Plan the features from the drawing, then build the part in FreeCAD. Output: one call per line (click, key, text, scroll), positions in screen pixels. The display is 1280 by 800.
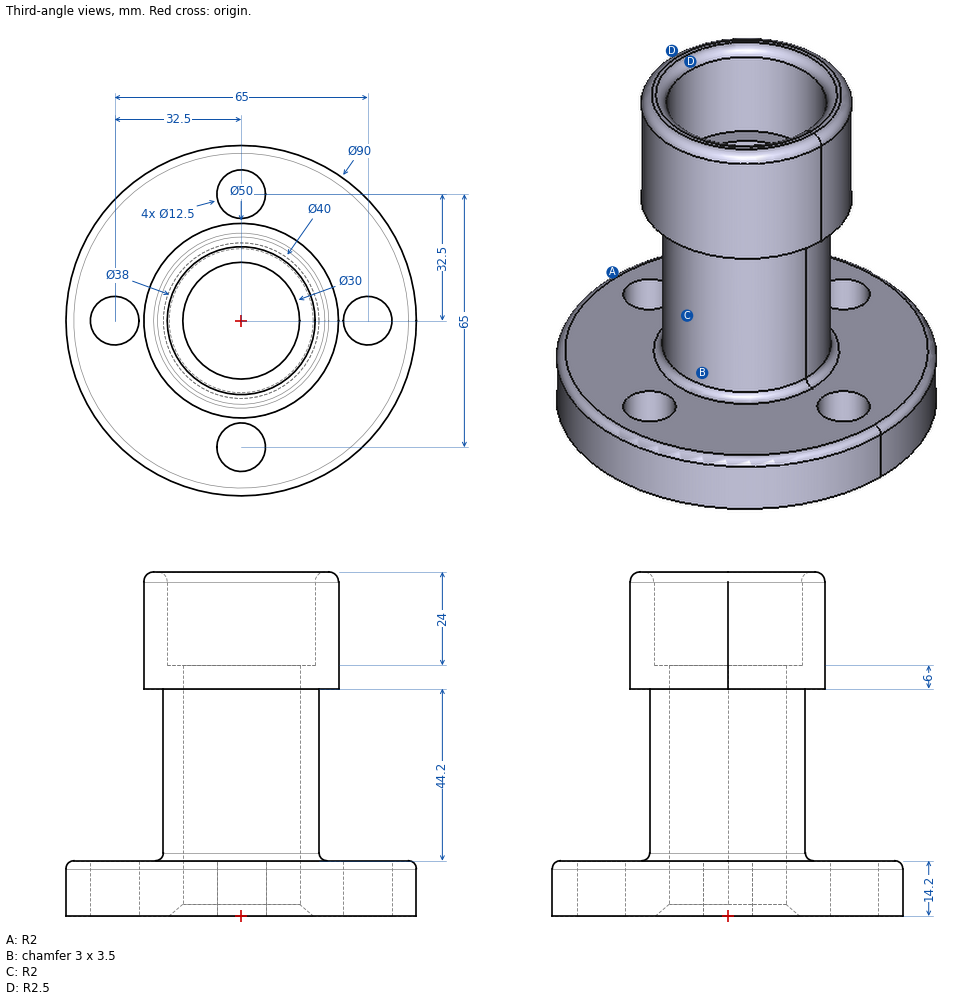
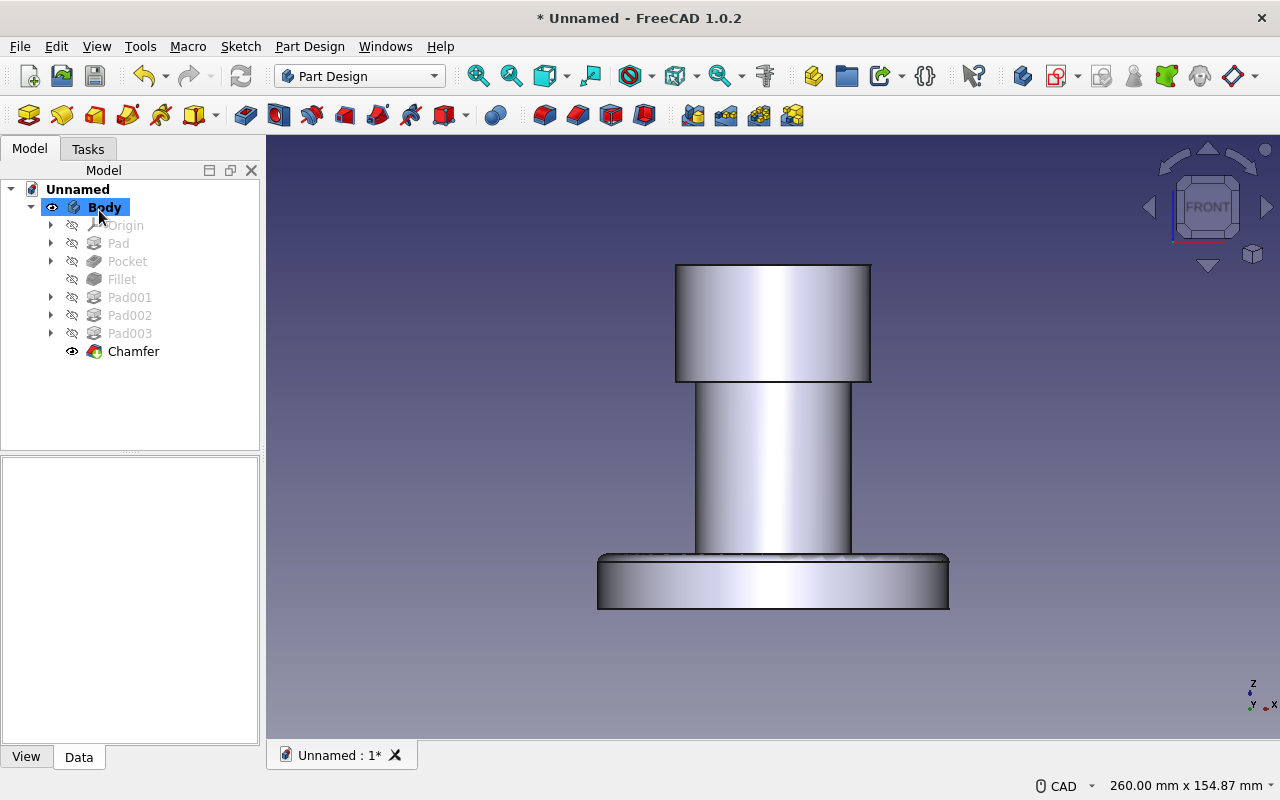
key(3)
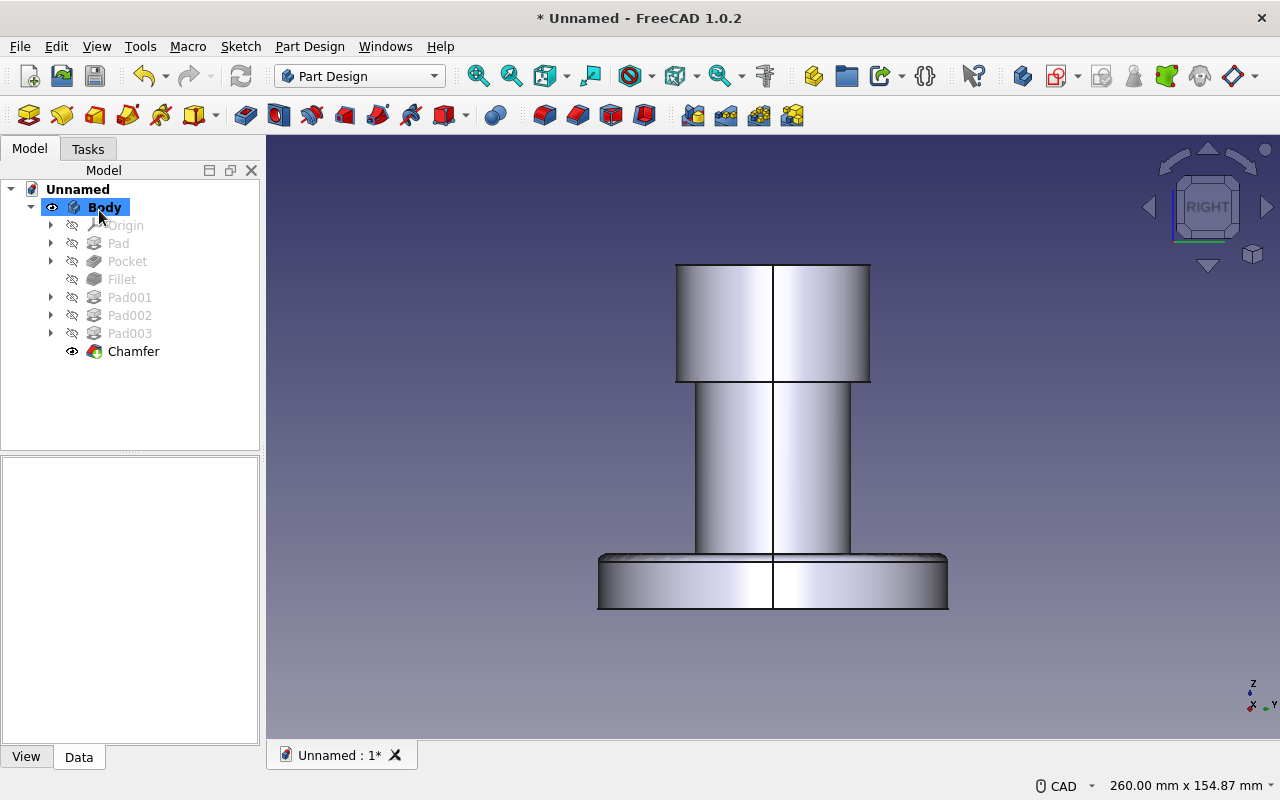
key(5)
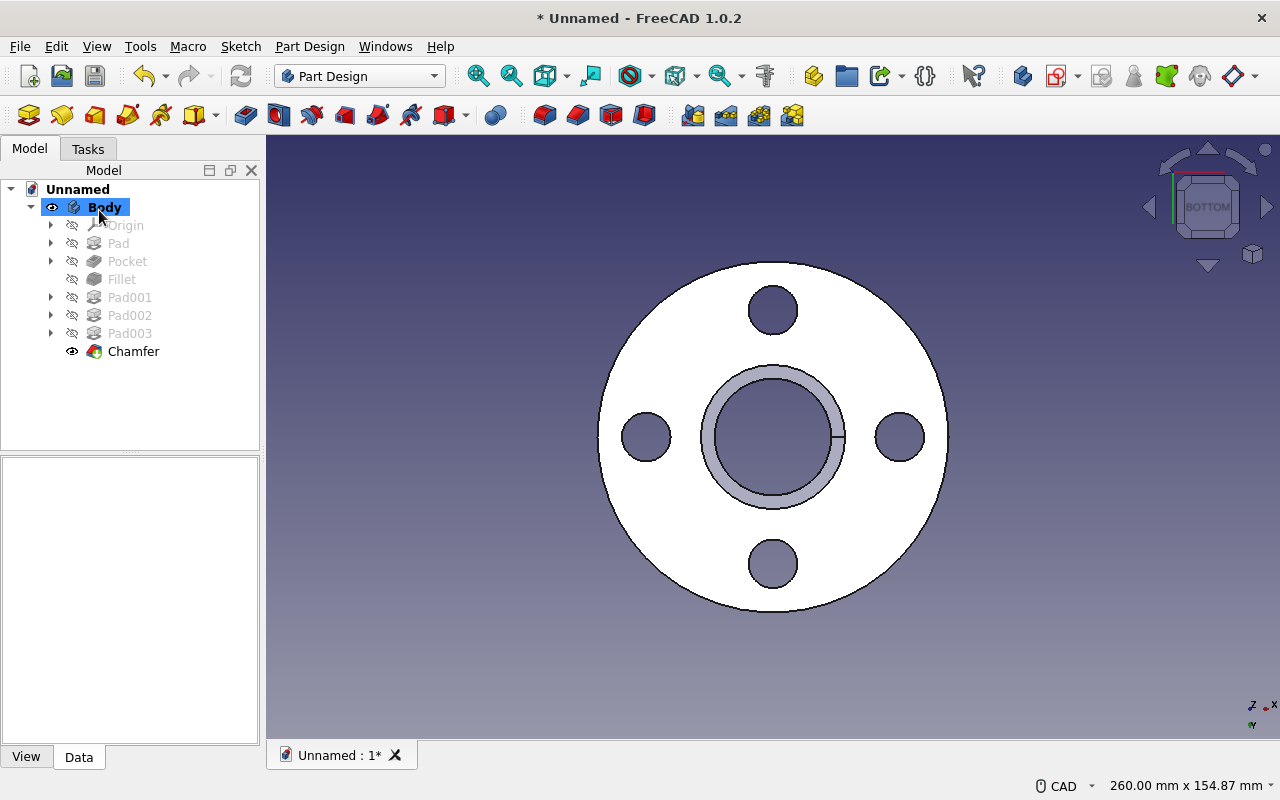
key(4)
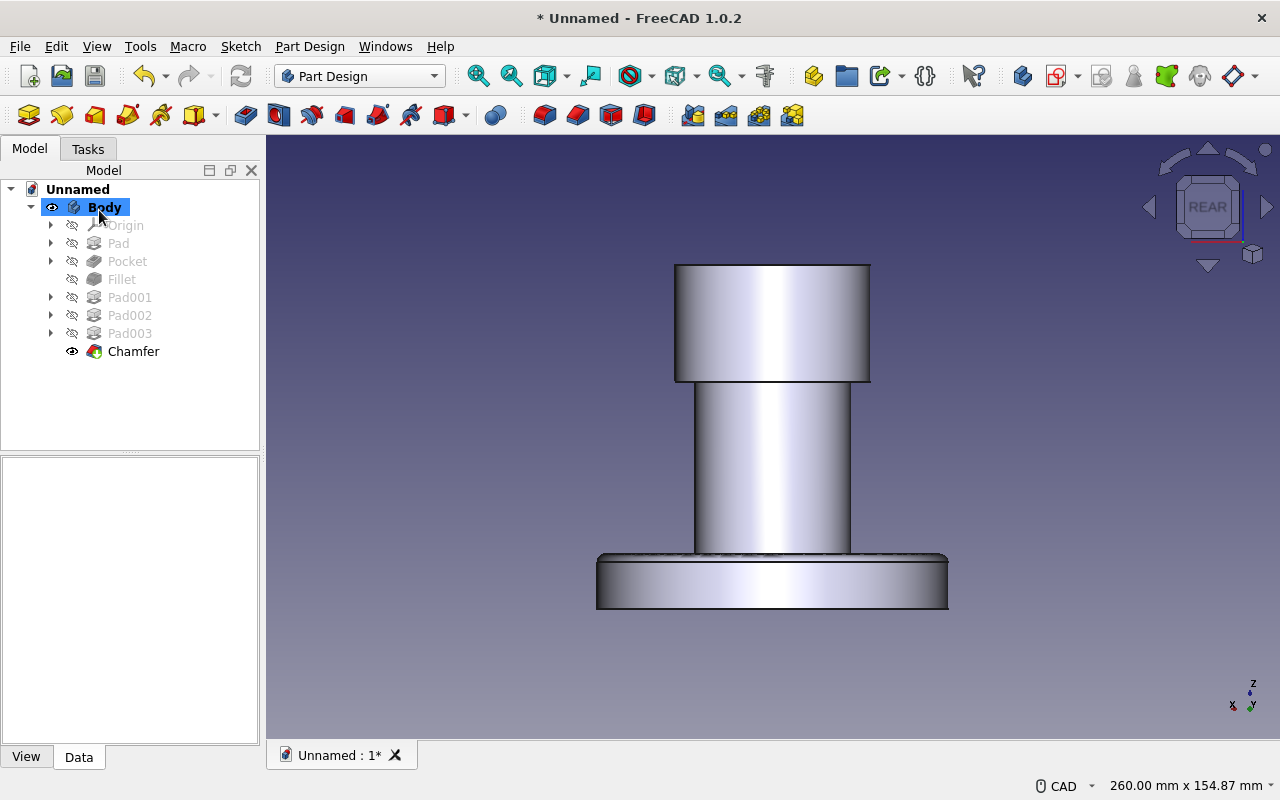
key(6)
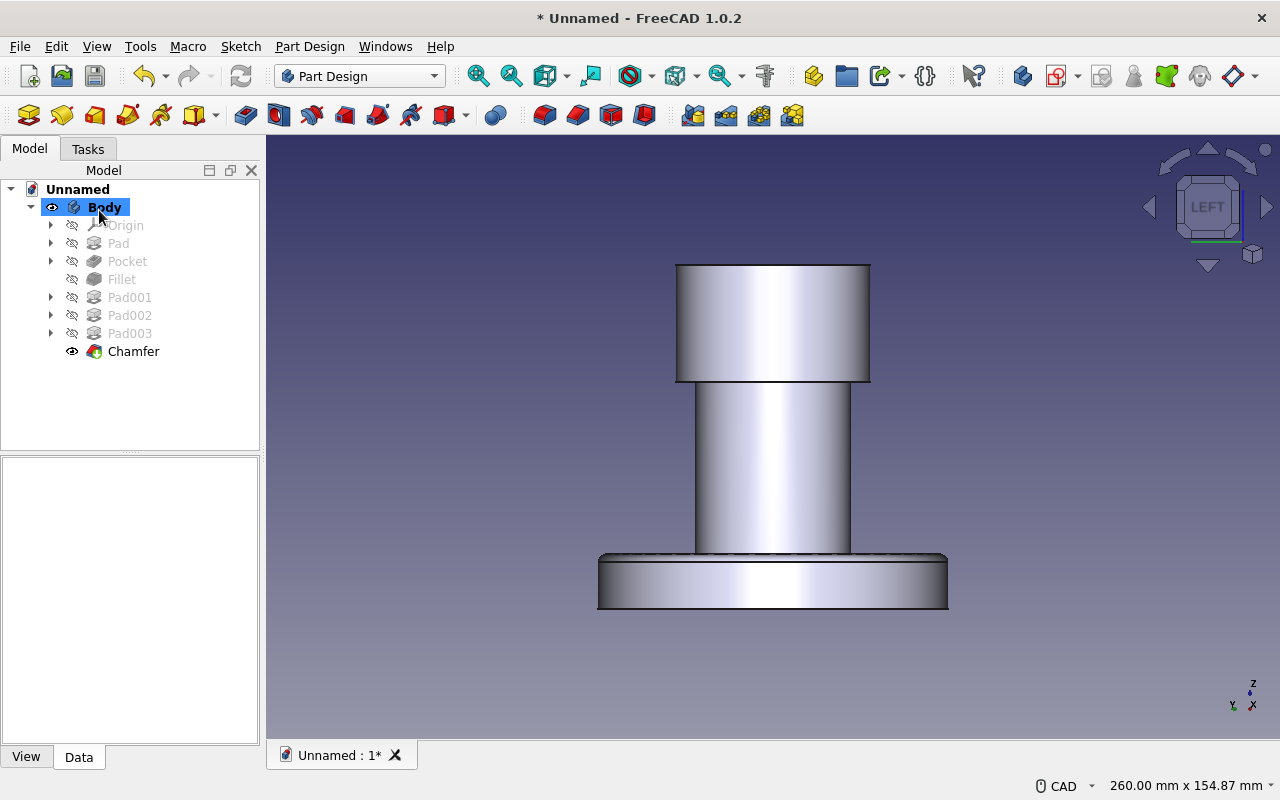
key(v)
key(3)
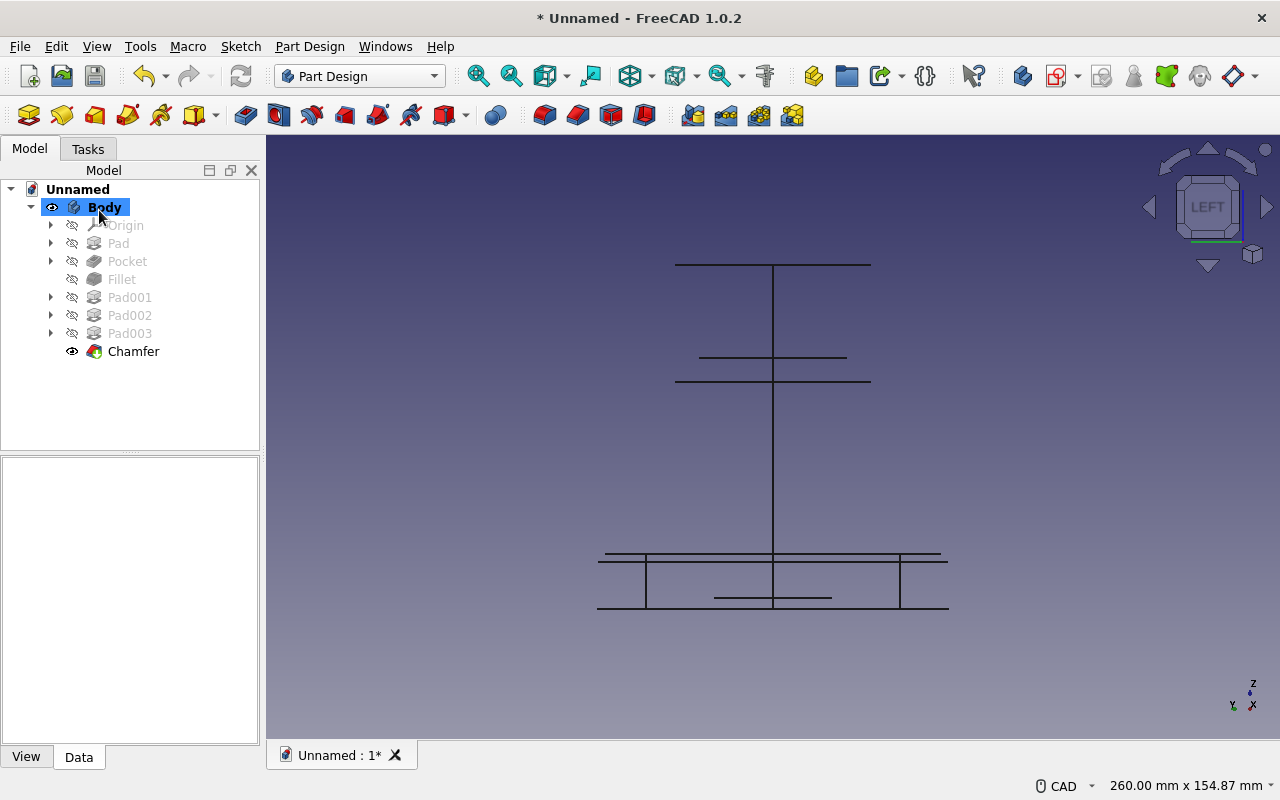
key(0)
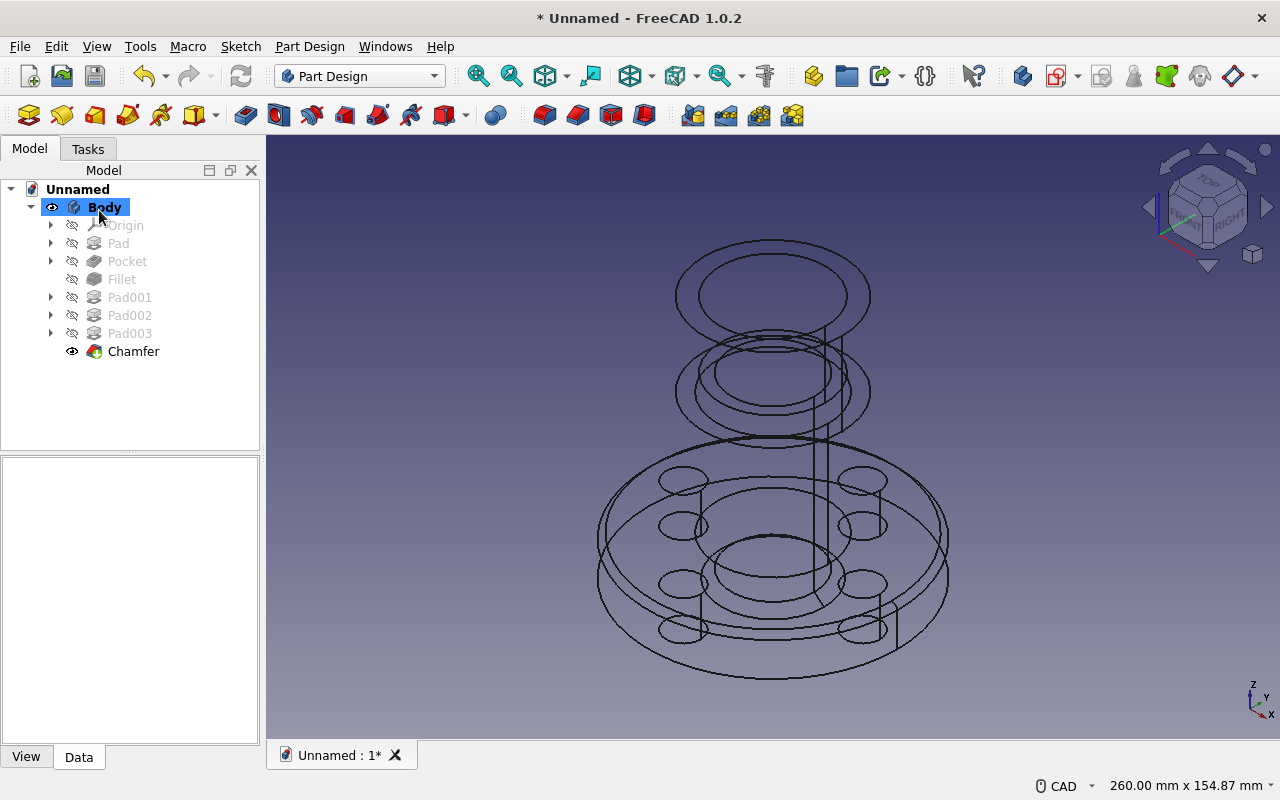
click(718, 500)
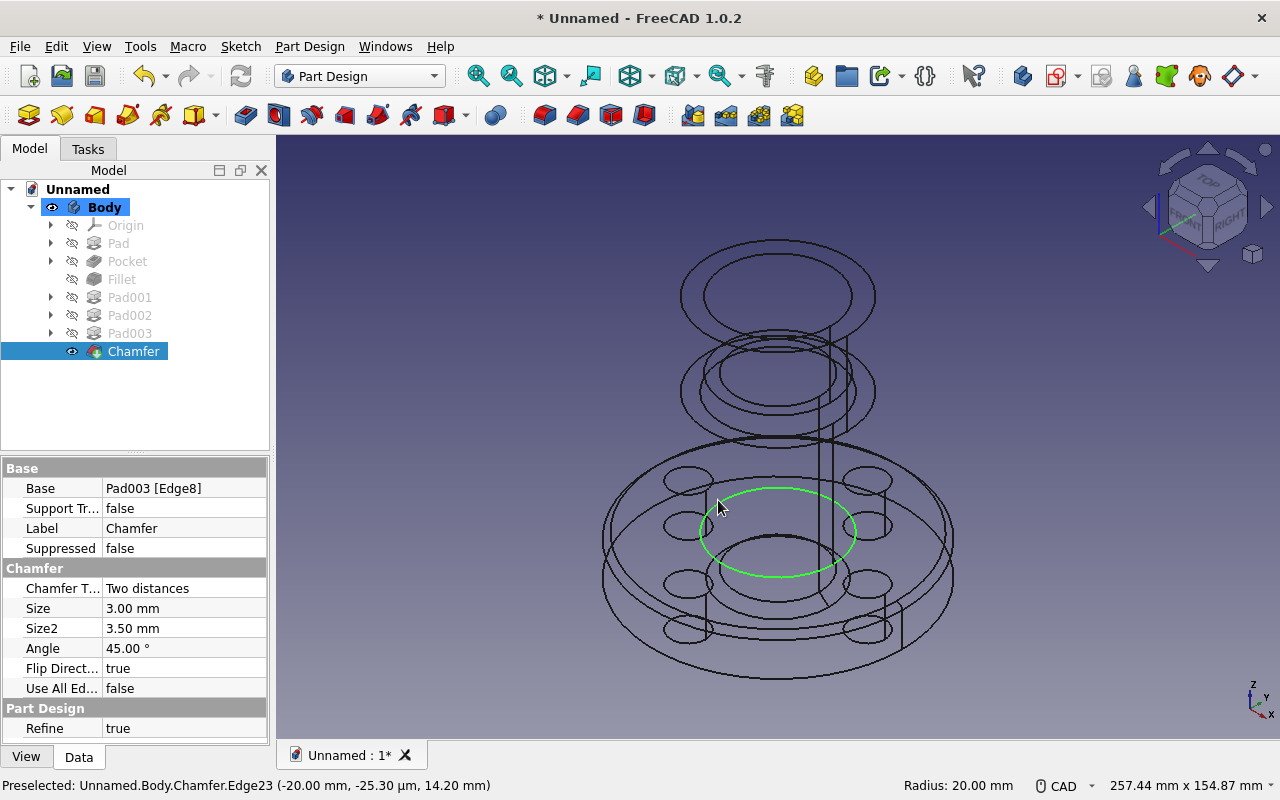
key(v)
key(1)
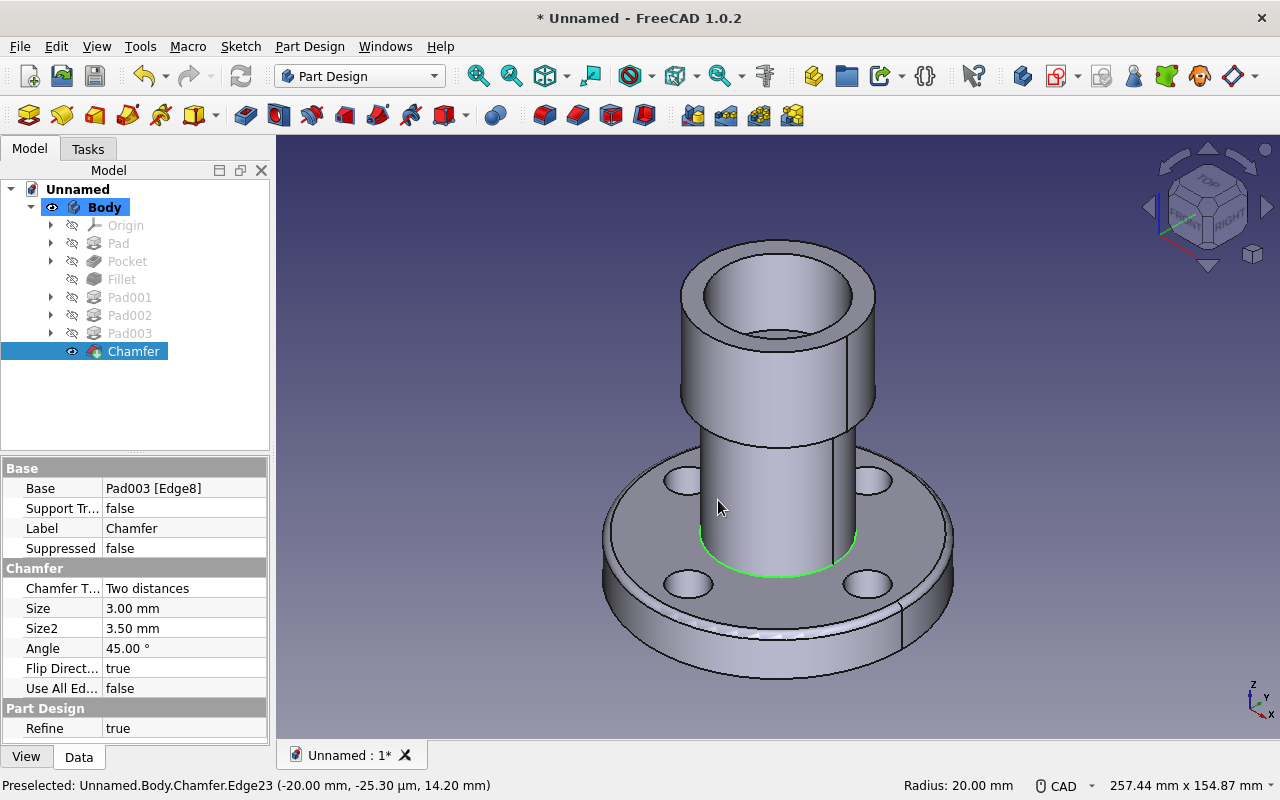
click(545, 116)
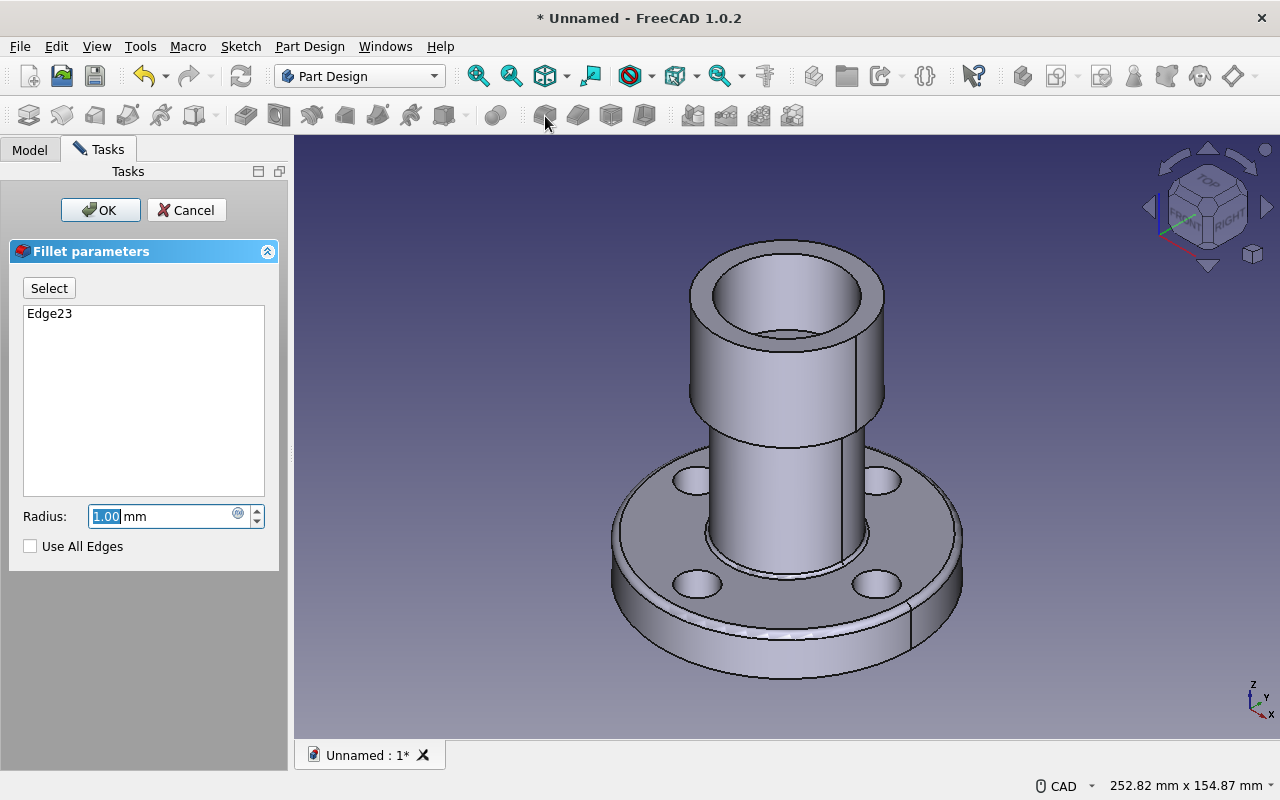
text(2)
key(Tab)